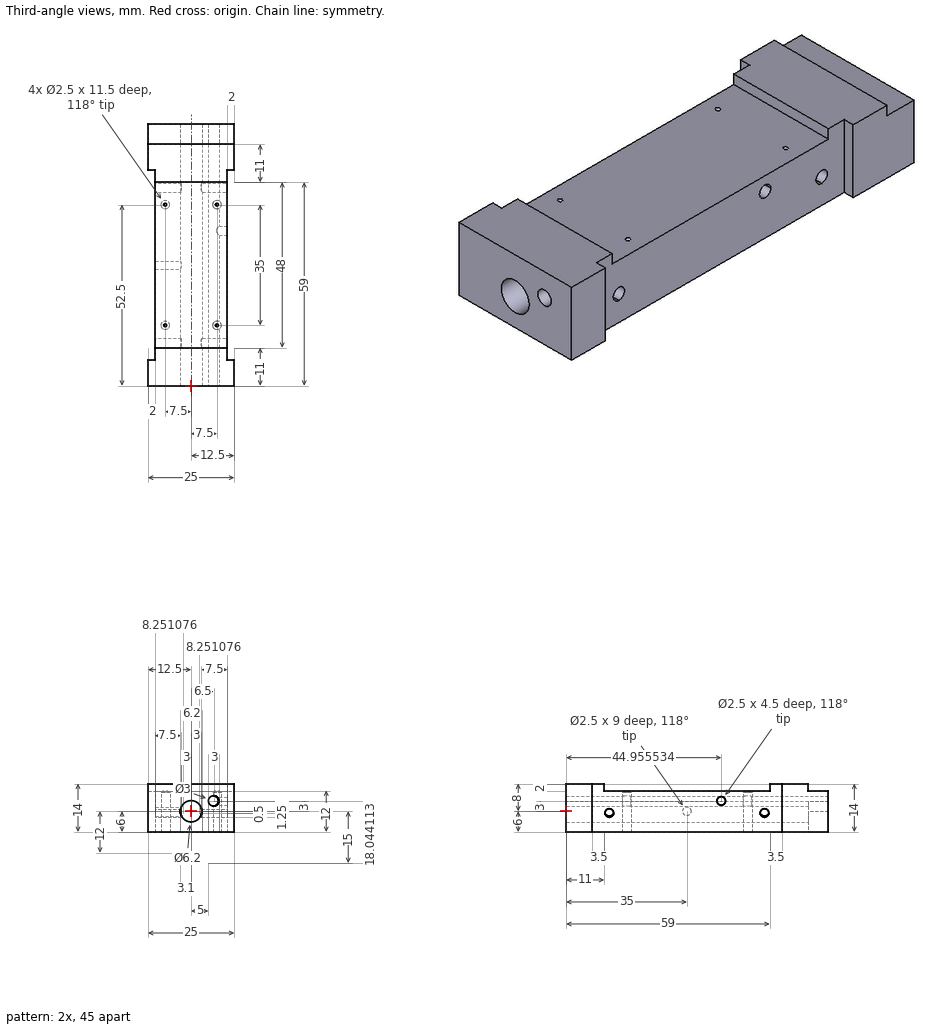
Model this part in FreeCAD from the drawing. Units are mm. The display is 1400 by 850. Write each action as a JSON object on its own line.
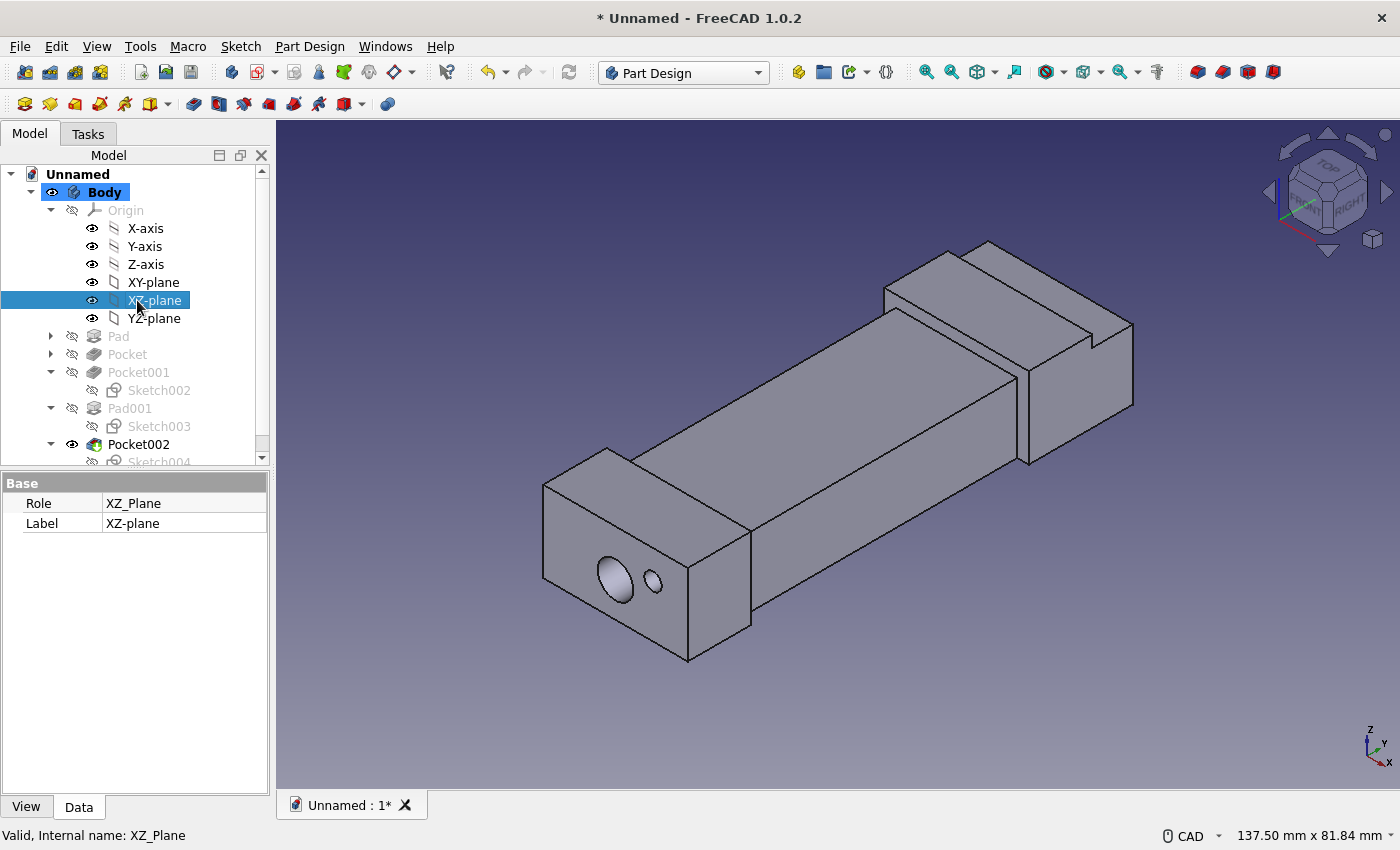
{"action": "left_click", "coordinate": [394, 72]}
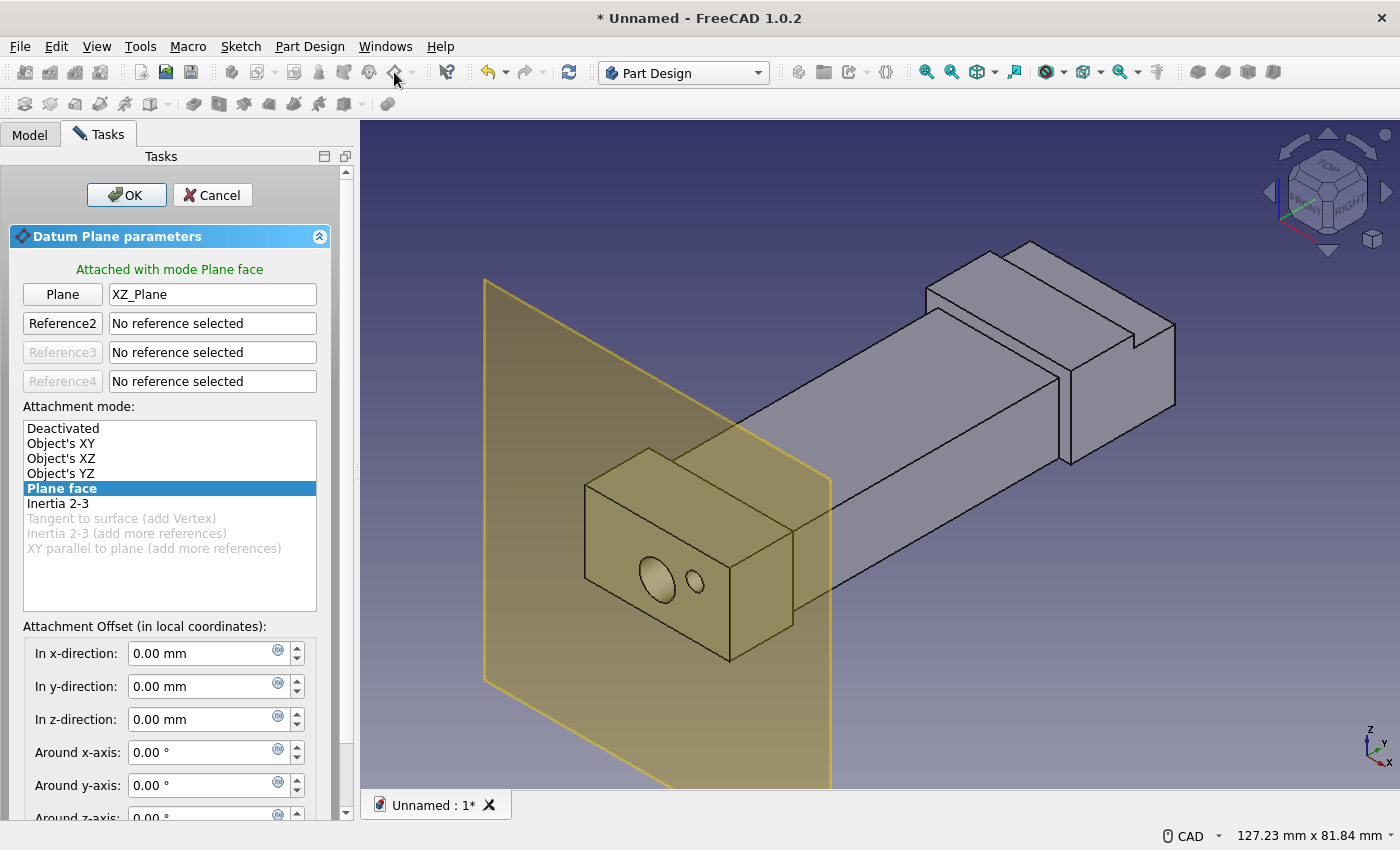
{"action": "triple_click", "coordinate": [210, 720]}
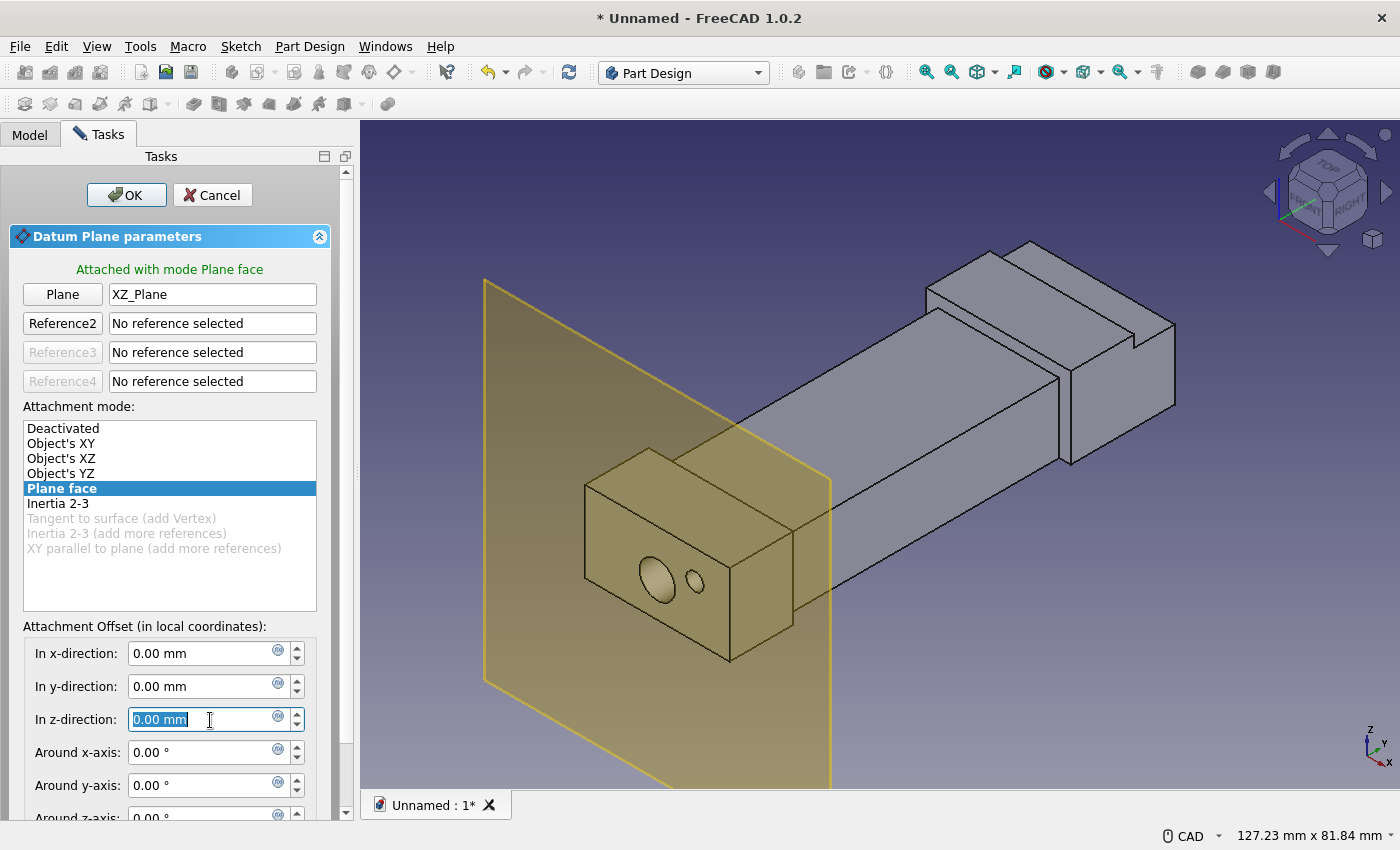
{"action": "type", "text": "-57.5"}
{"action": "key", "text": "Tab"}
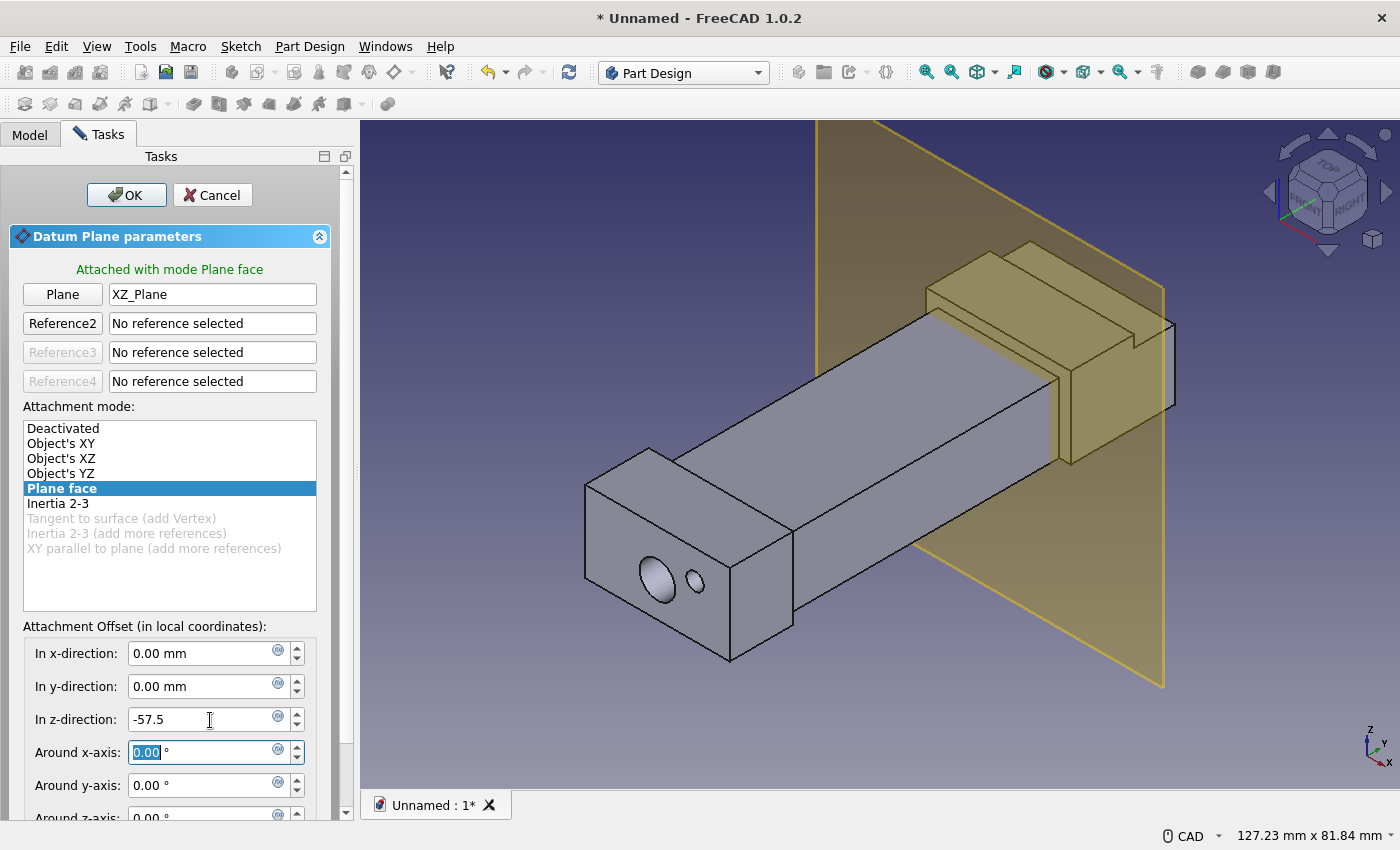
{"action": "left_click", "coordinate": [127, 195]}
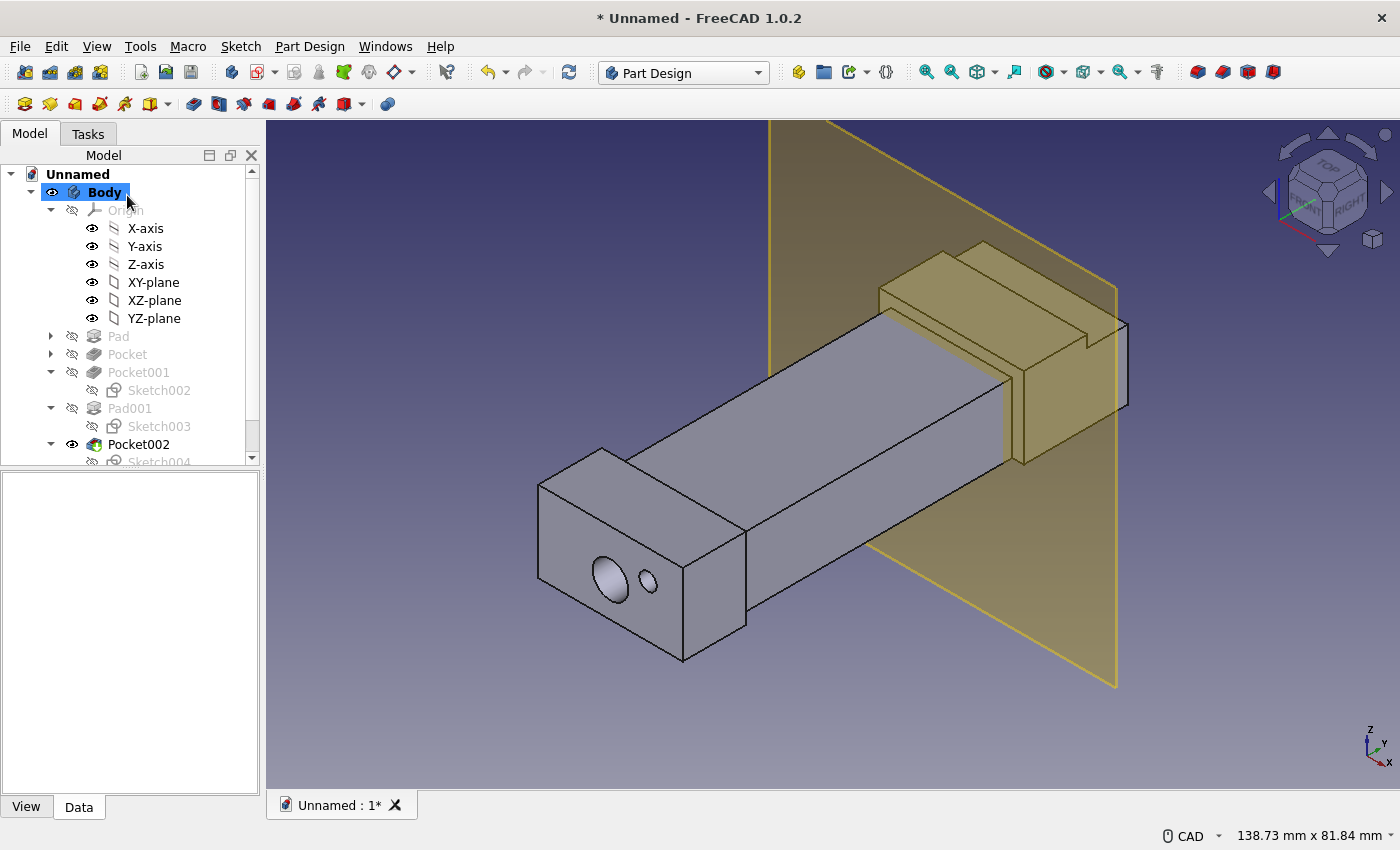
{"action": "scroll", "coordinate": [101, 314], "scroll_direction": "down", "scroll_amount": 3}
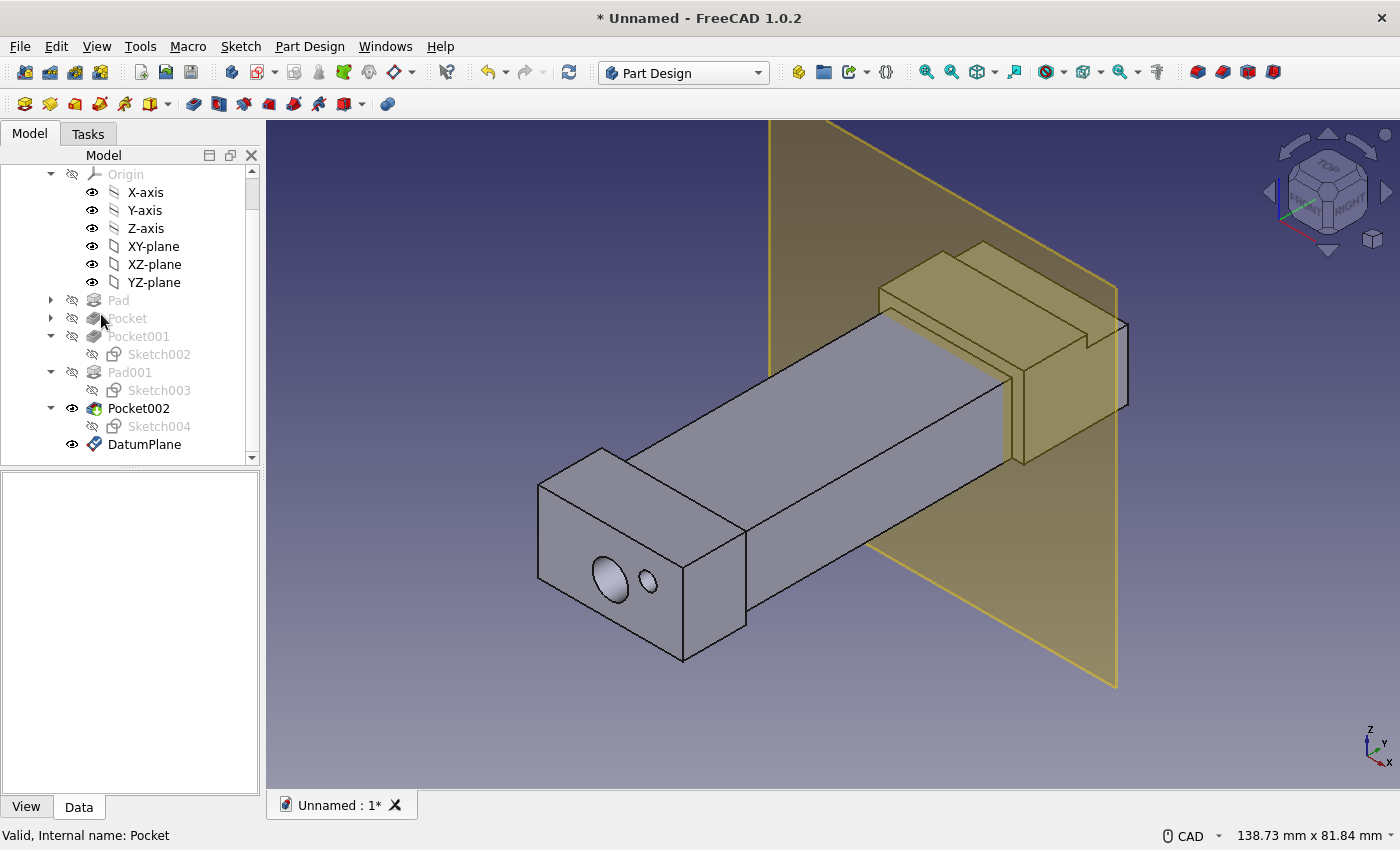
{"action": "left_click", "coordinate": [117, 444]}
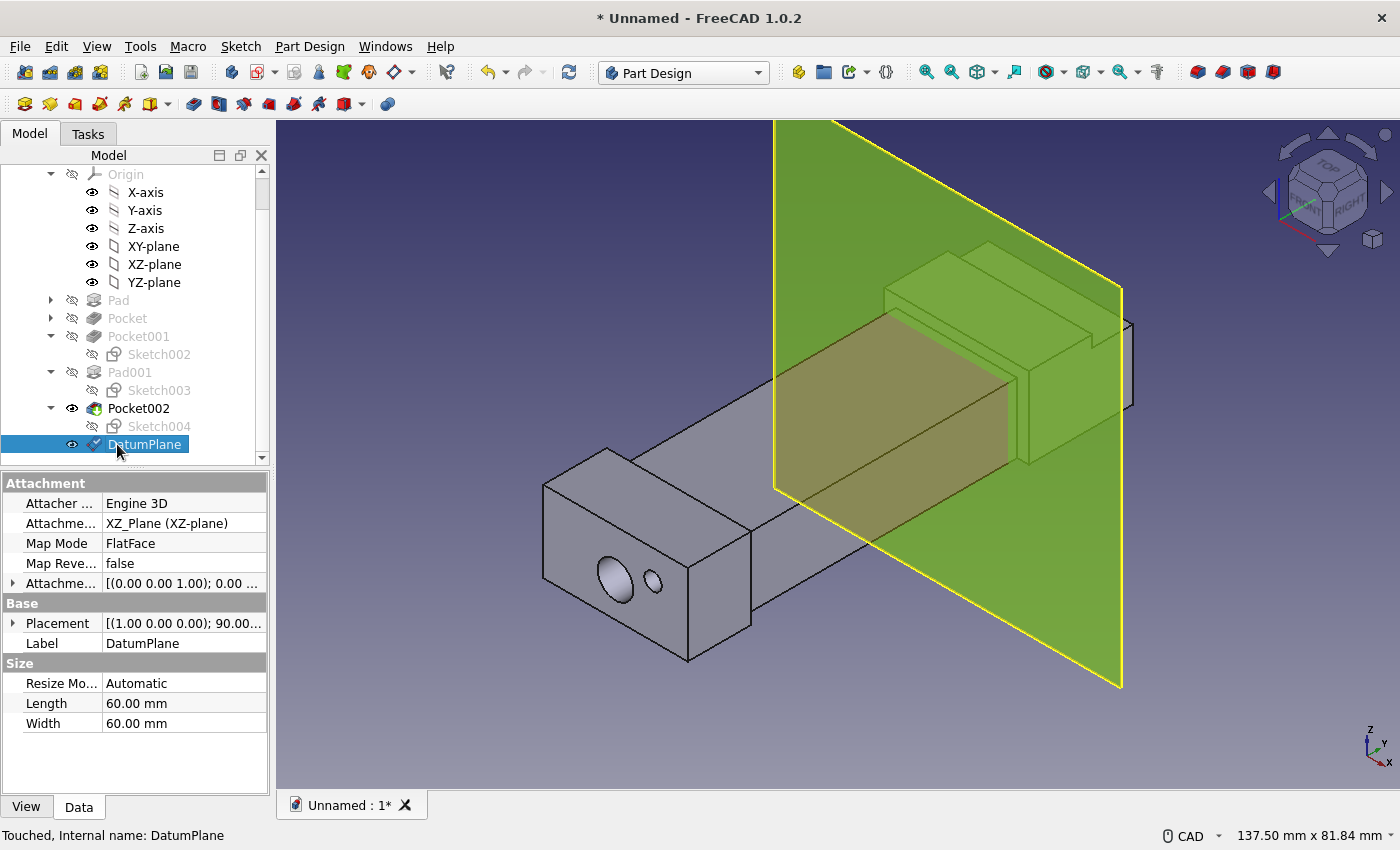
{"action": "left_click", "coordinate": [256, 72]}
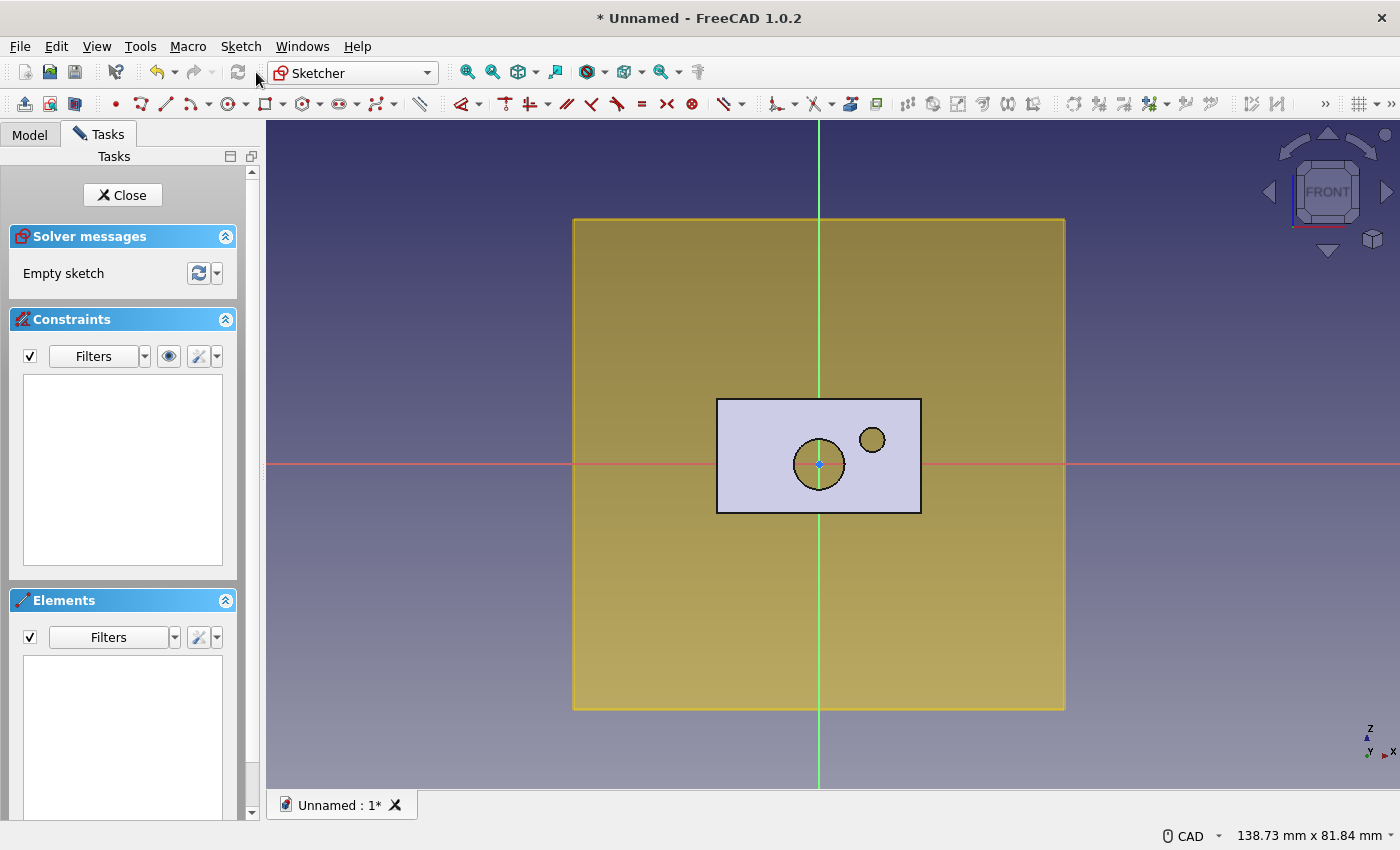
{"action": "left_click", "coordinate": [75, 104]}